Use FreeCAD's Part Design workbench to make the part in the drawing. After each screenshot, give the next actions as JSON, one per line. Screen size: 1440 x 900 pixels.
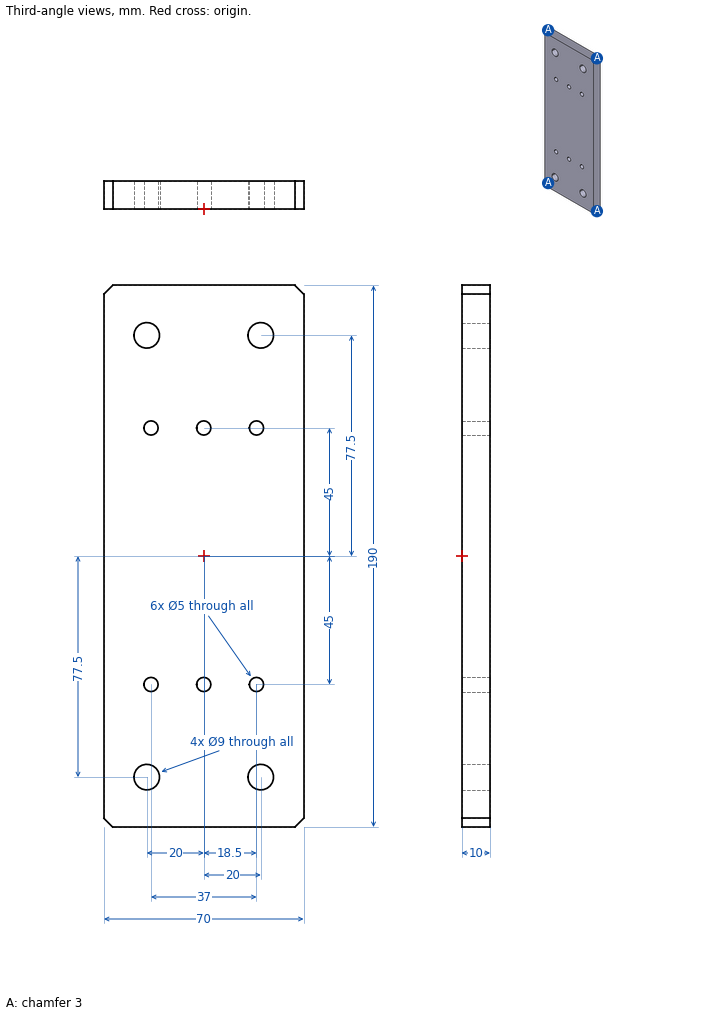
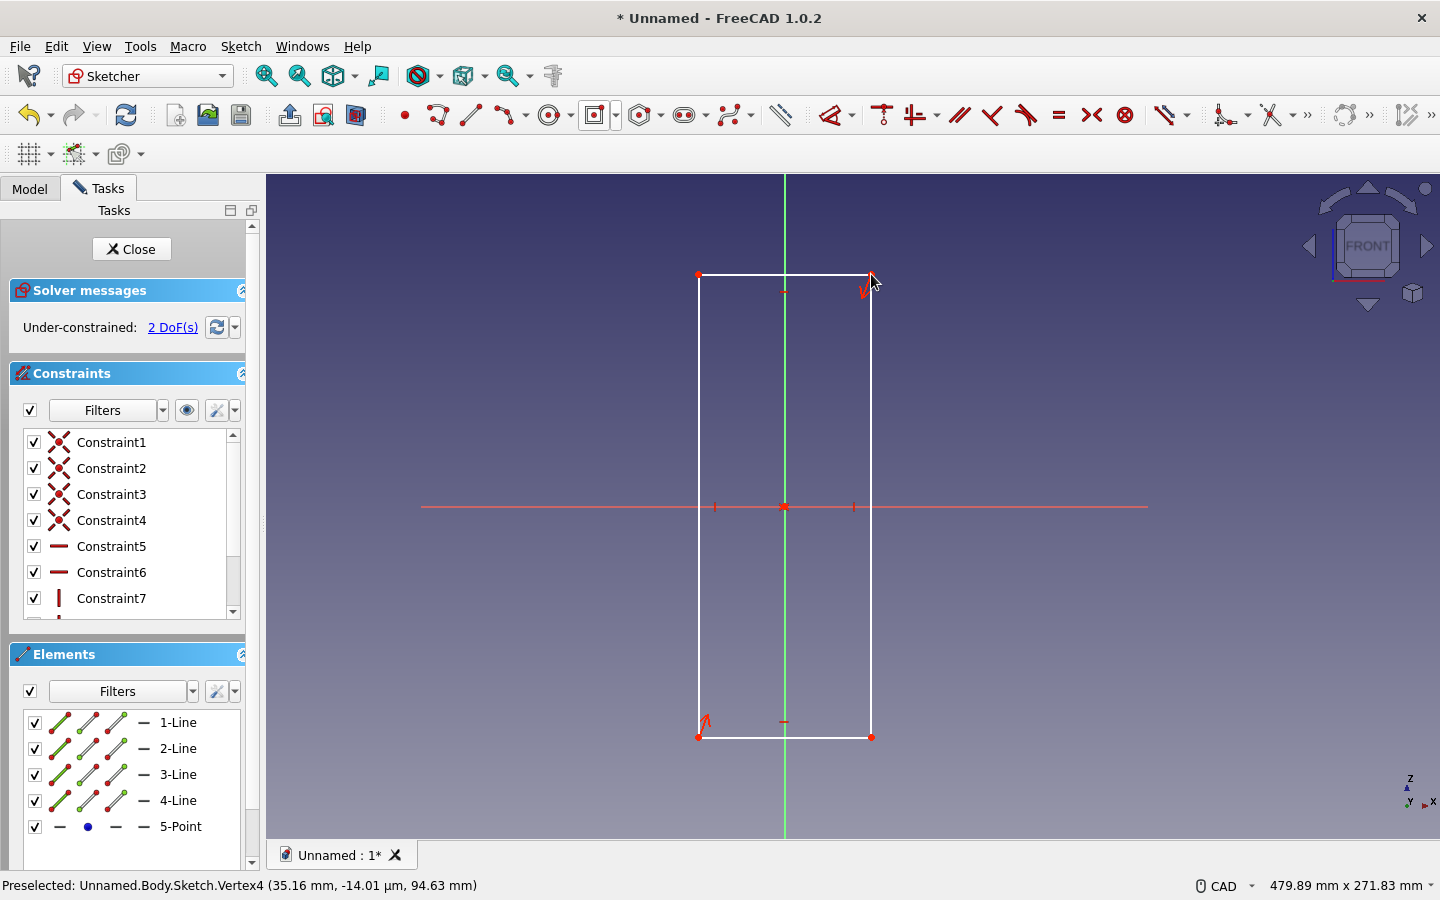
{"action": "left_click", "coordinate": [751, 738]}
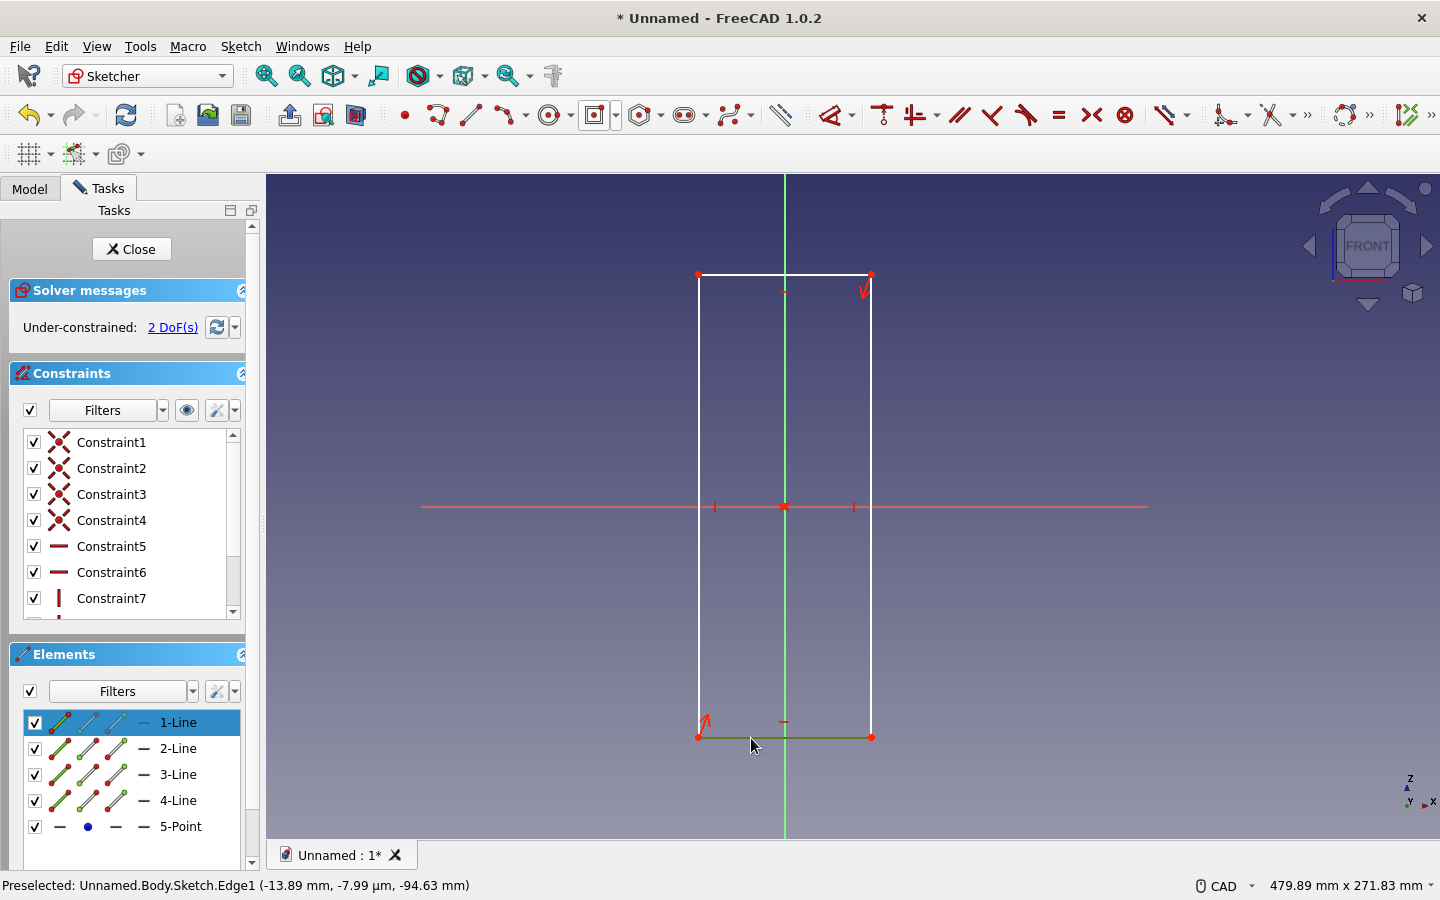
{"action": "left_click", "coordinate": [852, 116]}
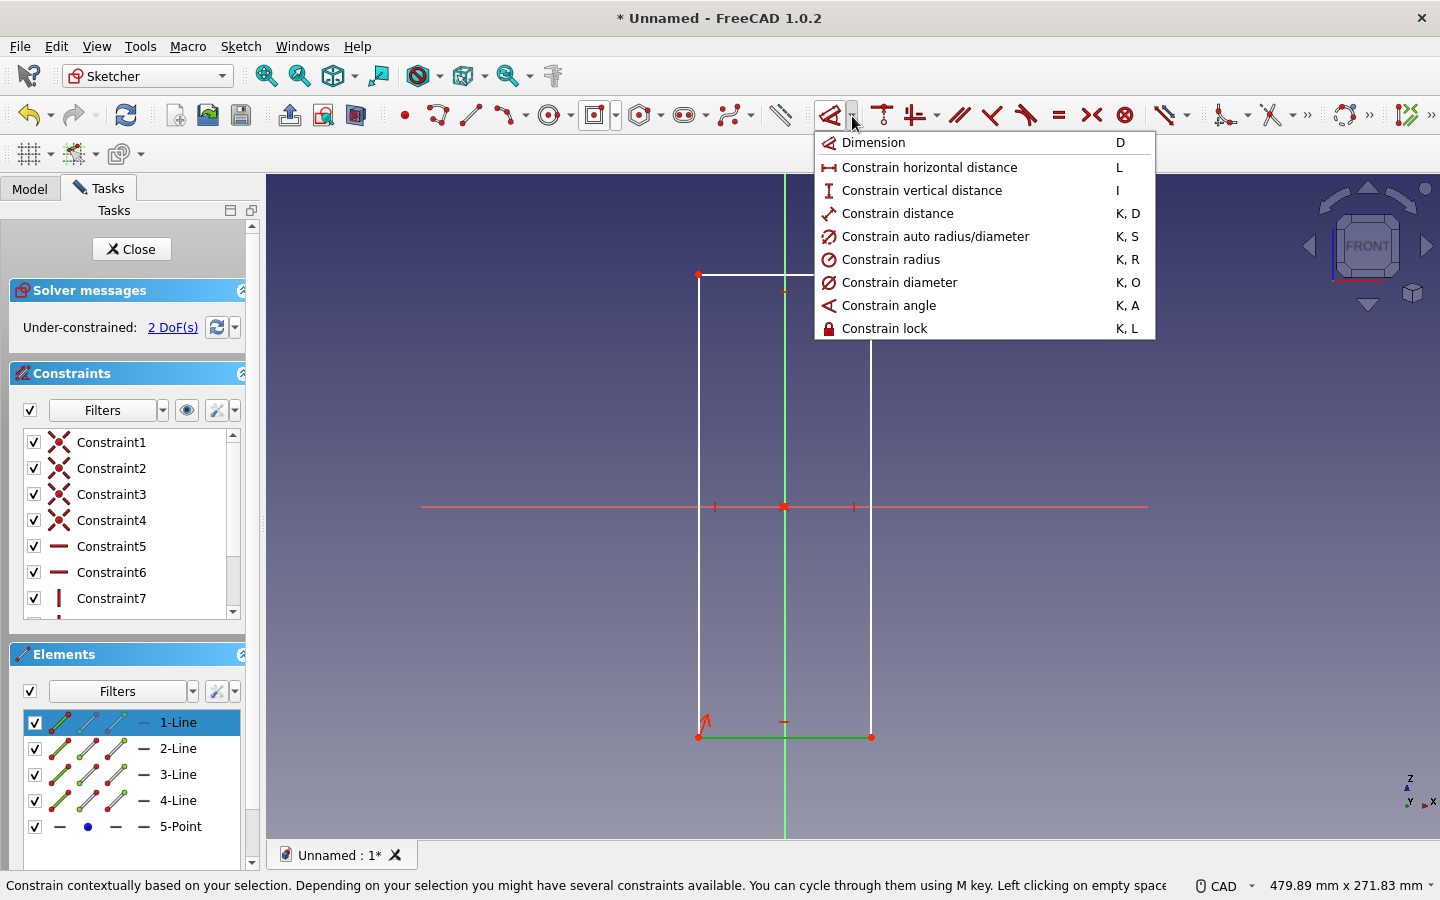
{"action": "left_click", "coordinate": [985, 168]}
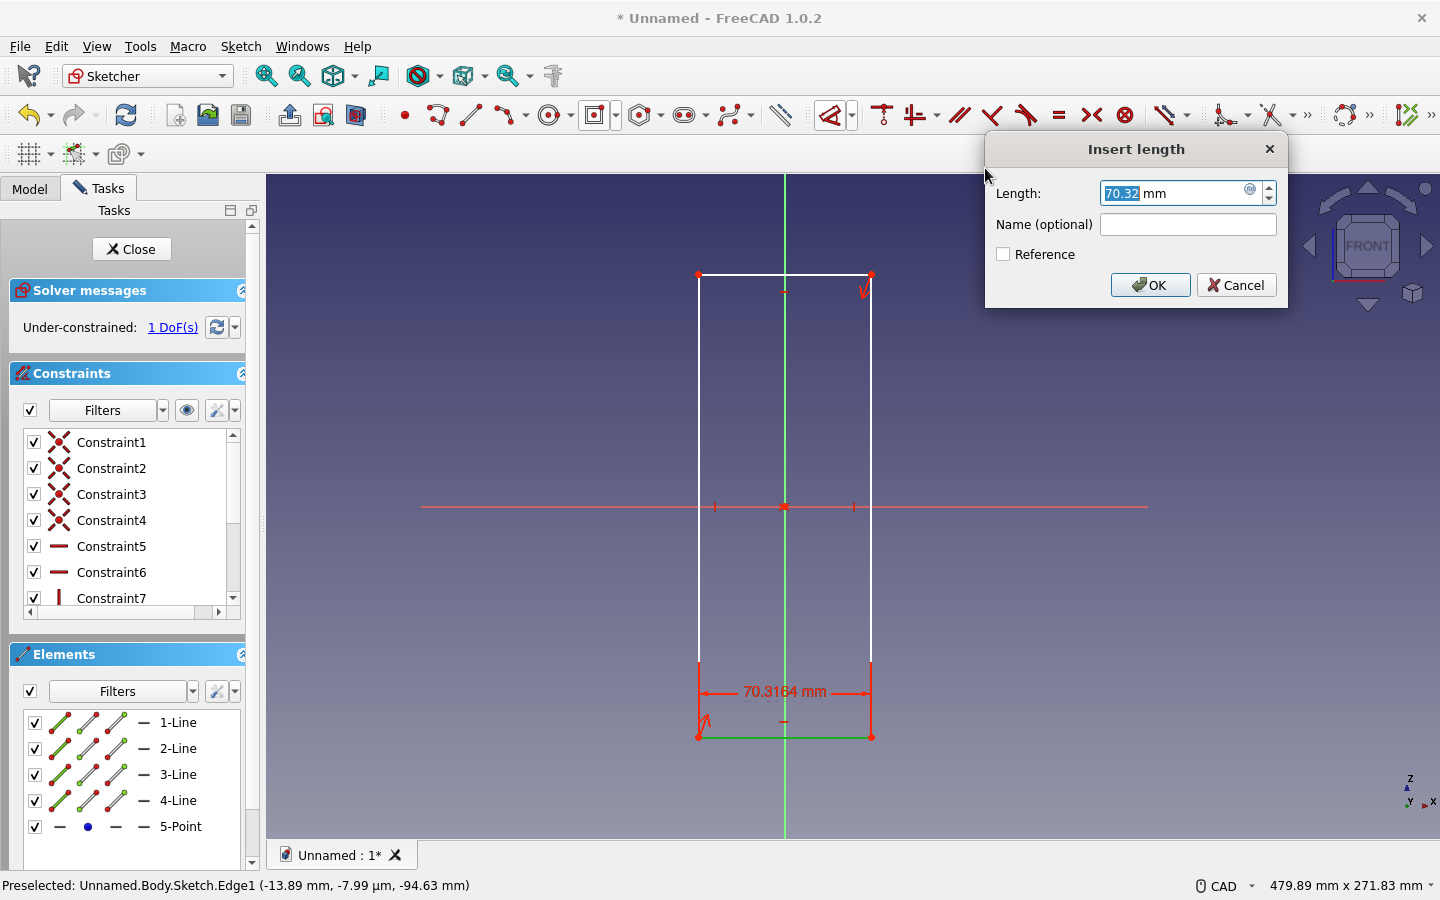
{"action": "type", "text": "70"}
{"action": "key", "text": "Return"}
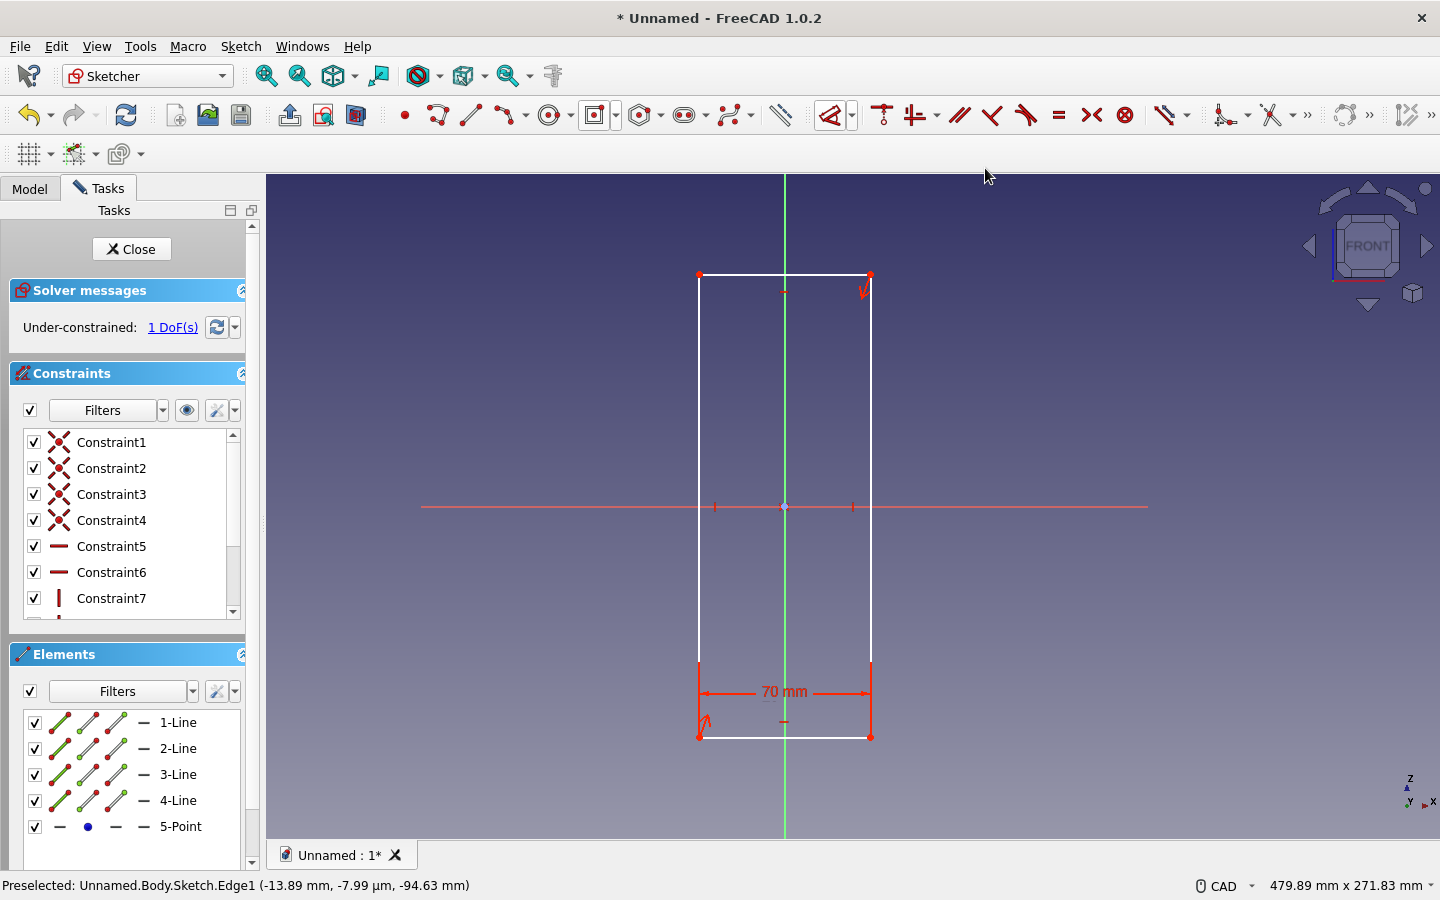
{"action": "left_click", "coordinate": [871, 599]}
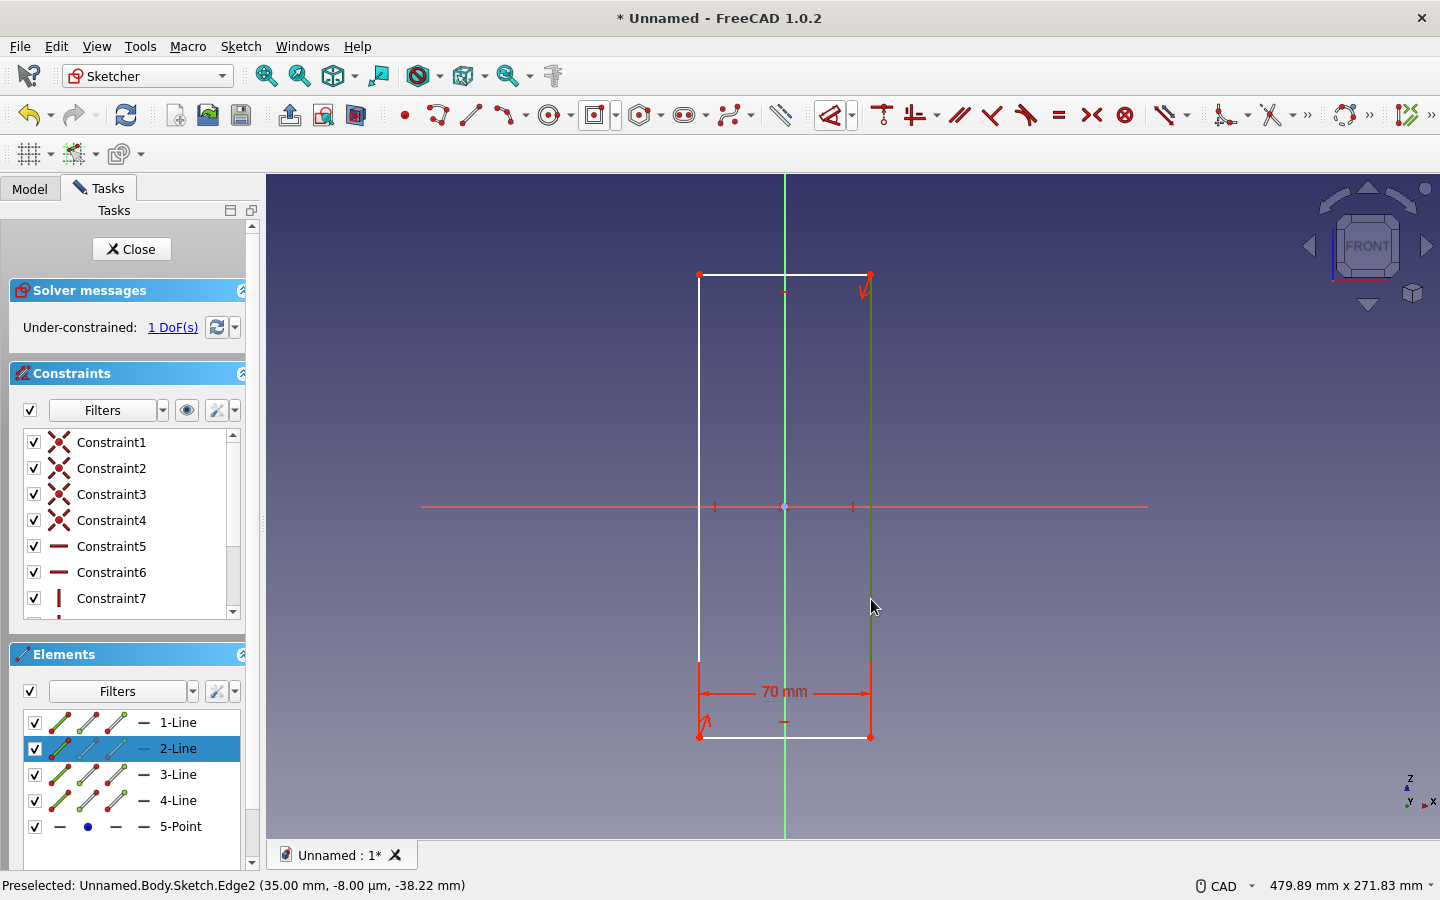
{"action": "key", "text": "i"}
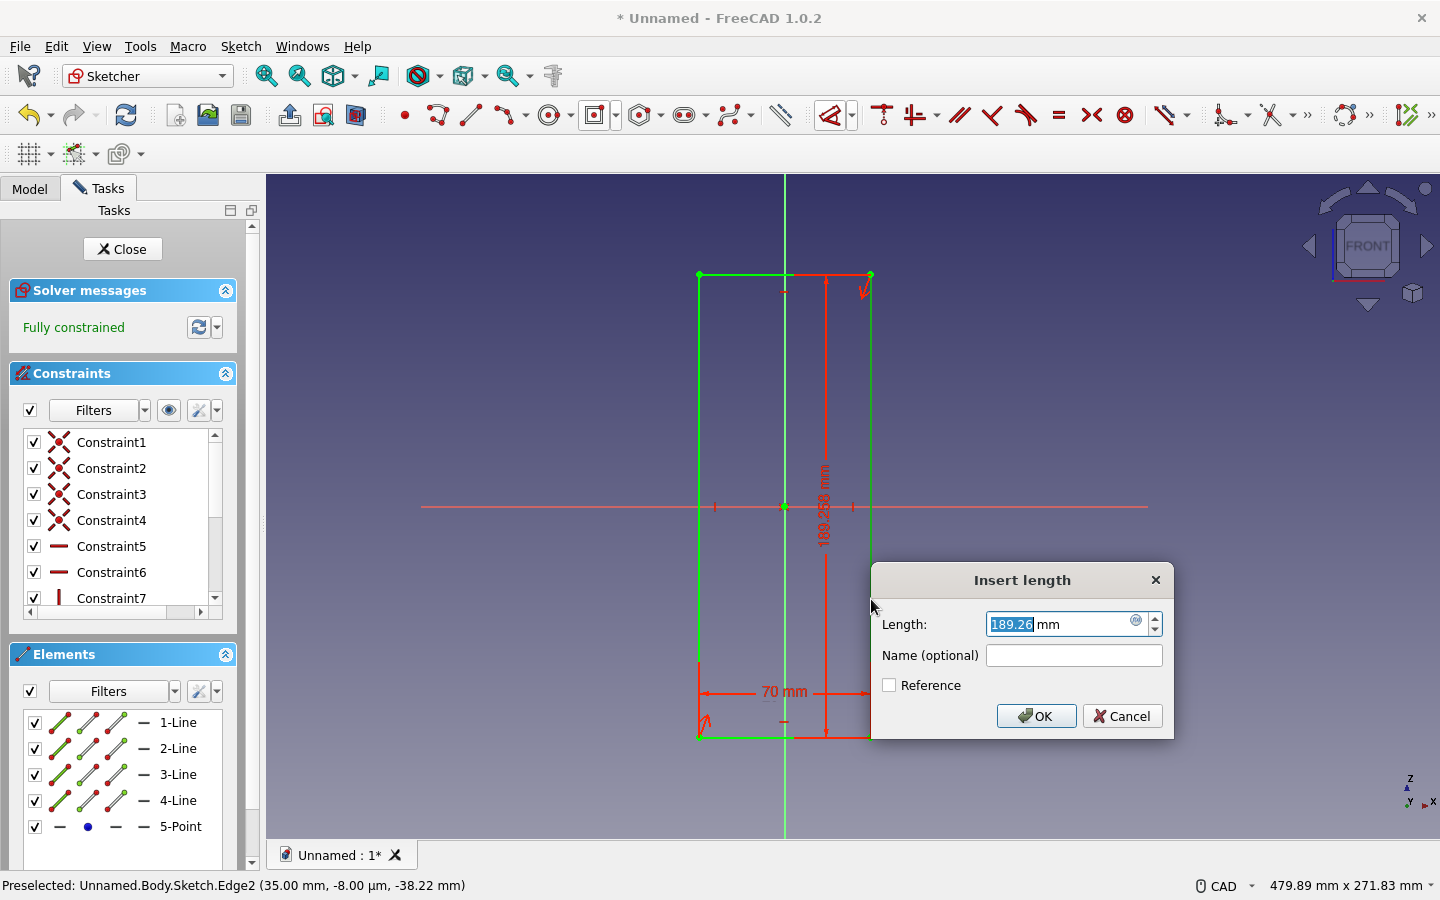
{"action": "type", "text": "190"}
{"action": "key", "text": "Return"}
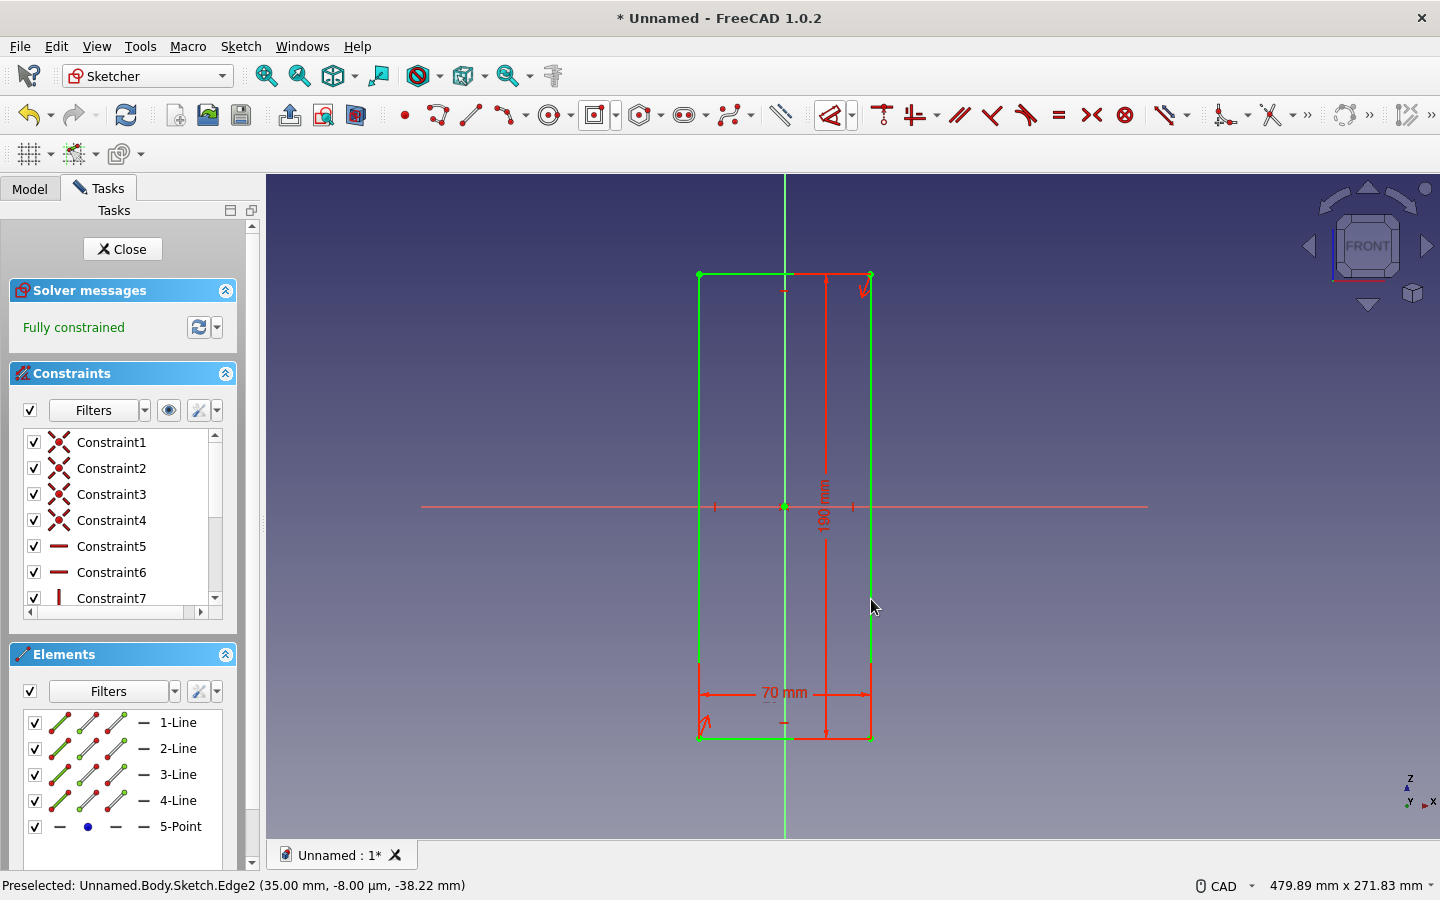
{"action": "left_click", "coordinate": [123, 249]}